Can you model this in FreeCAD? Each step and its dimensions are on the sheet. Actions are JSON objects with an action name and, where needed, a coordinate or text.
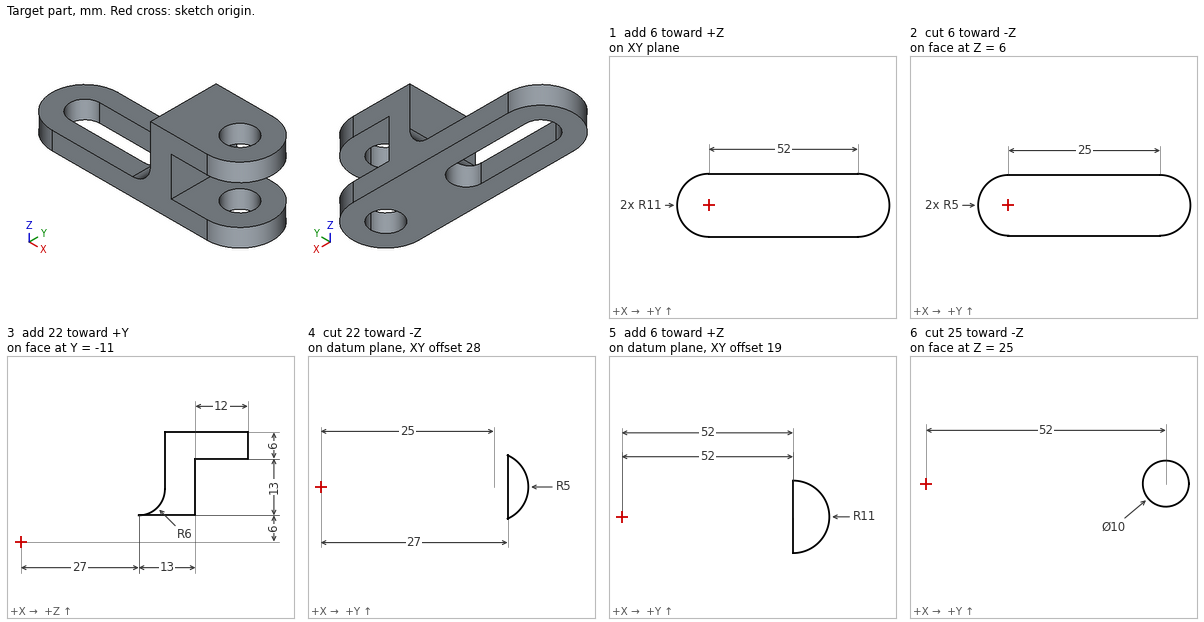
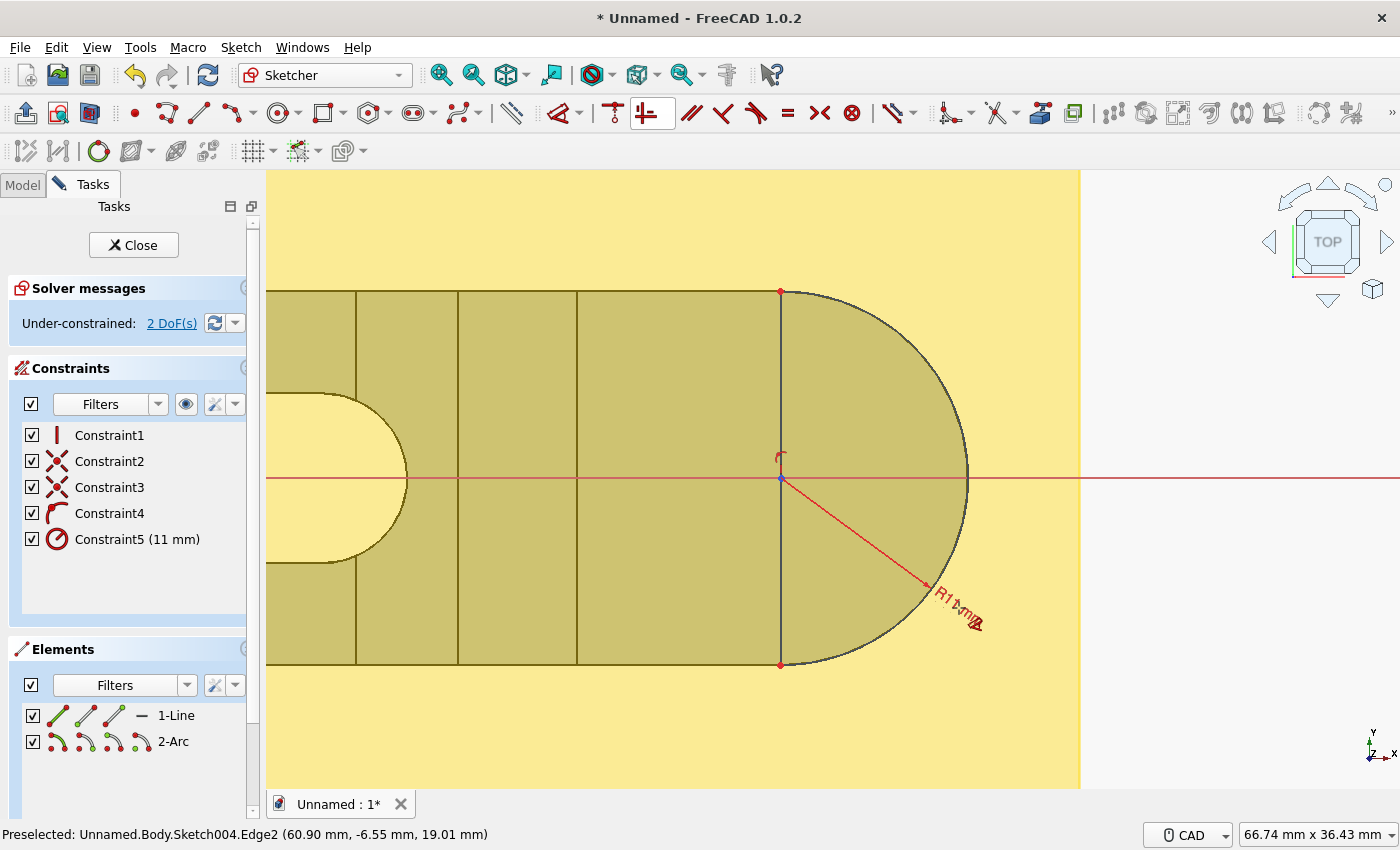
{"action": "left_click", "coordinate": [781, 291]}
{"action": "left_click", "coordinate": [537, 257]}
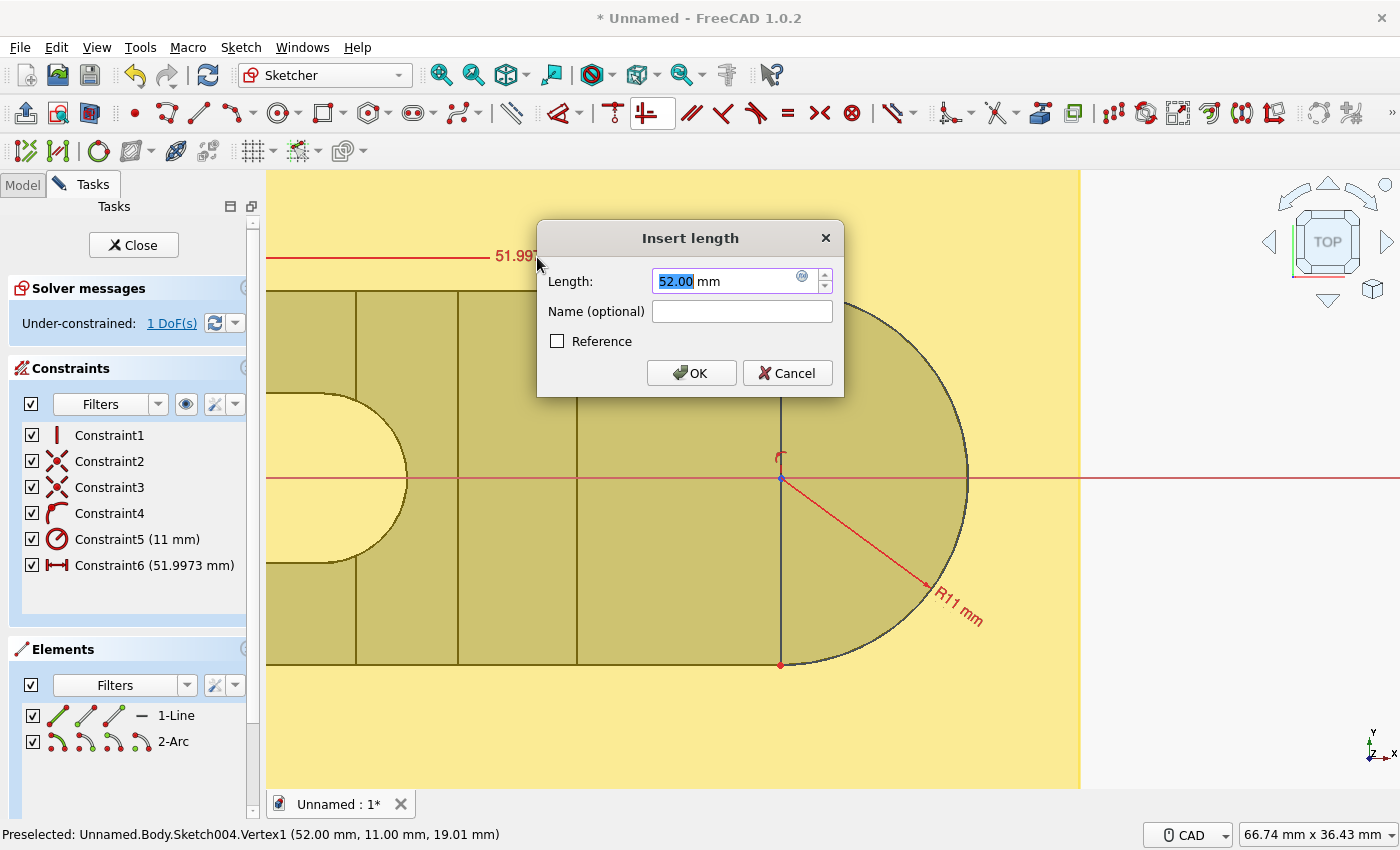
{"action": "type", "text": "52"}
{"action": "key", "text": "Return"}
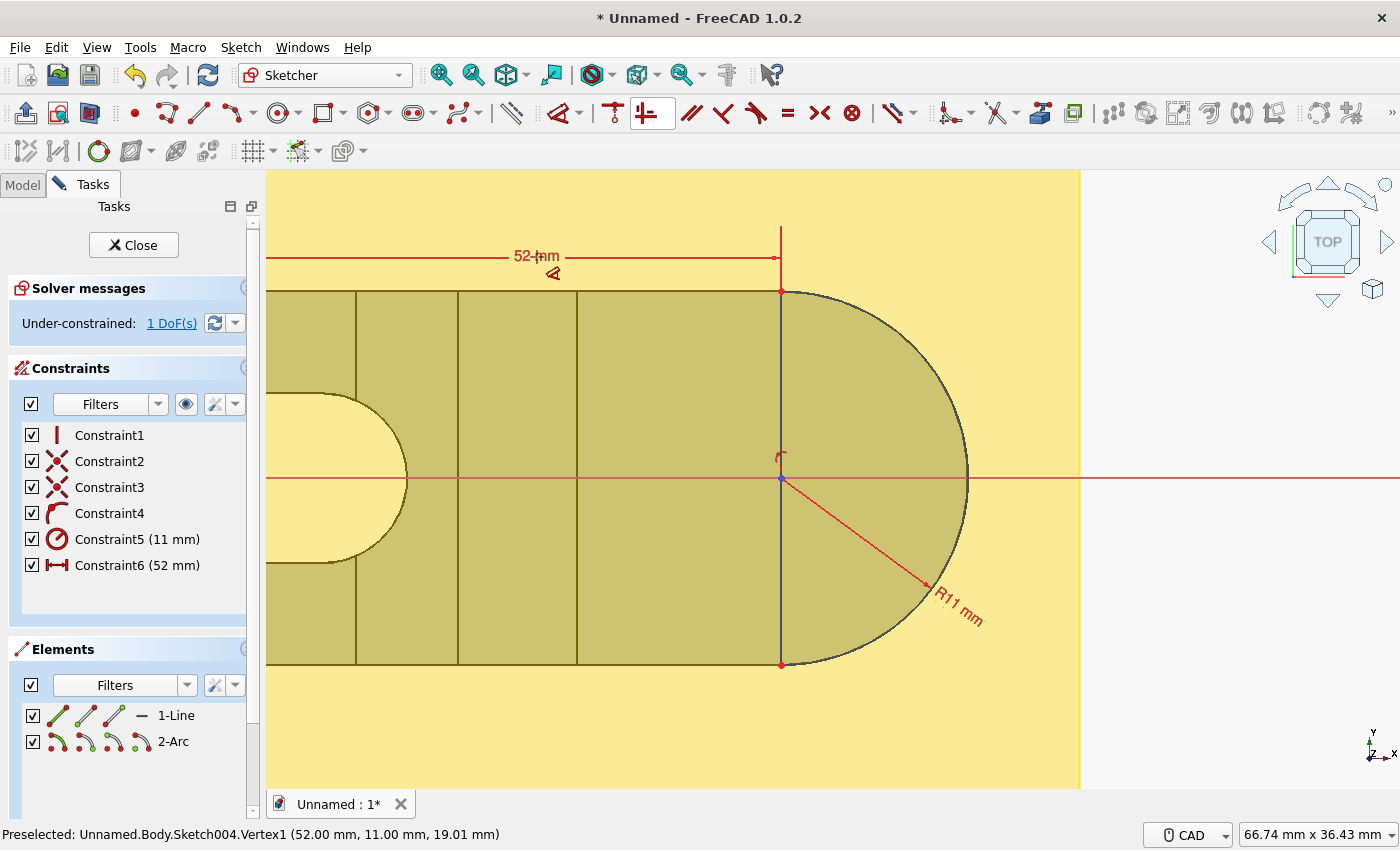
{"action": "left_click", "coordinate": [781, 478]}
{"action": "left_click", "coordinate": [538, 512]}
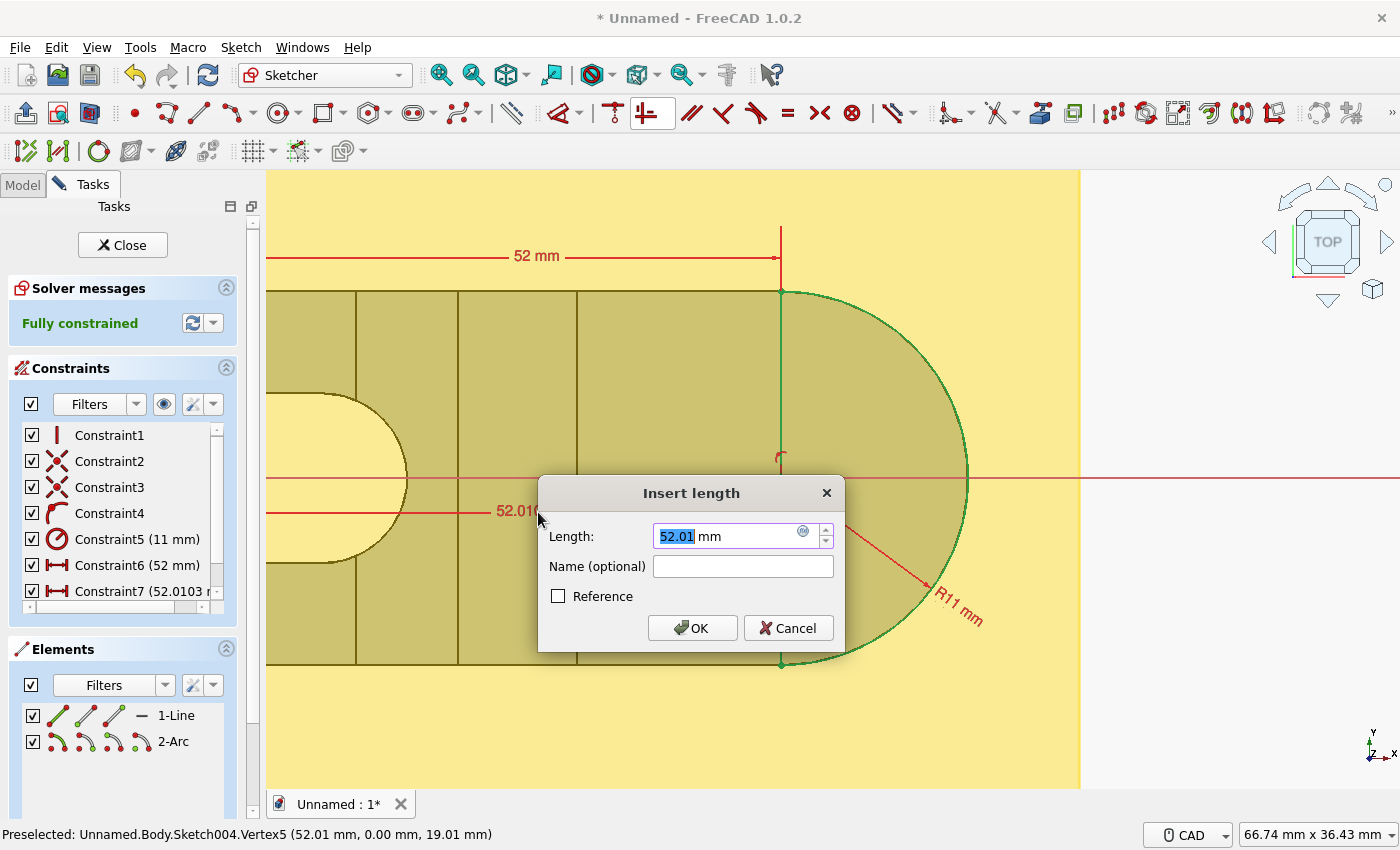
{"action": "type", "text": "52"}
{"action": "key", "text": "Return"}
{"action": "key", "text": "Escape"}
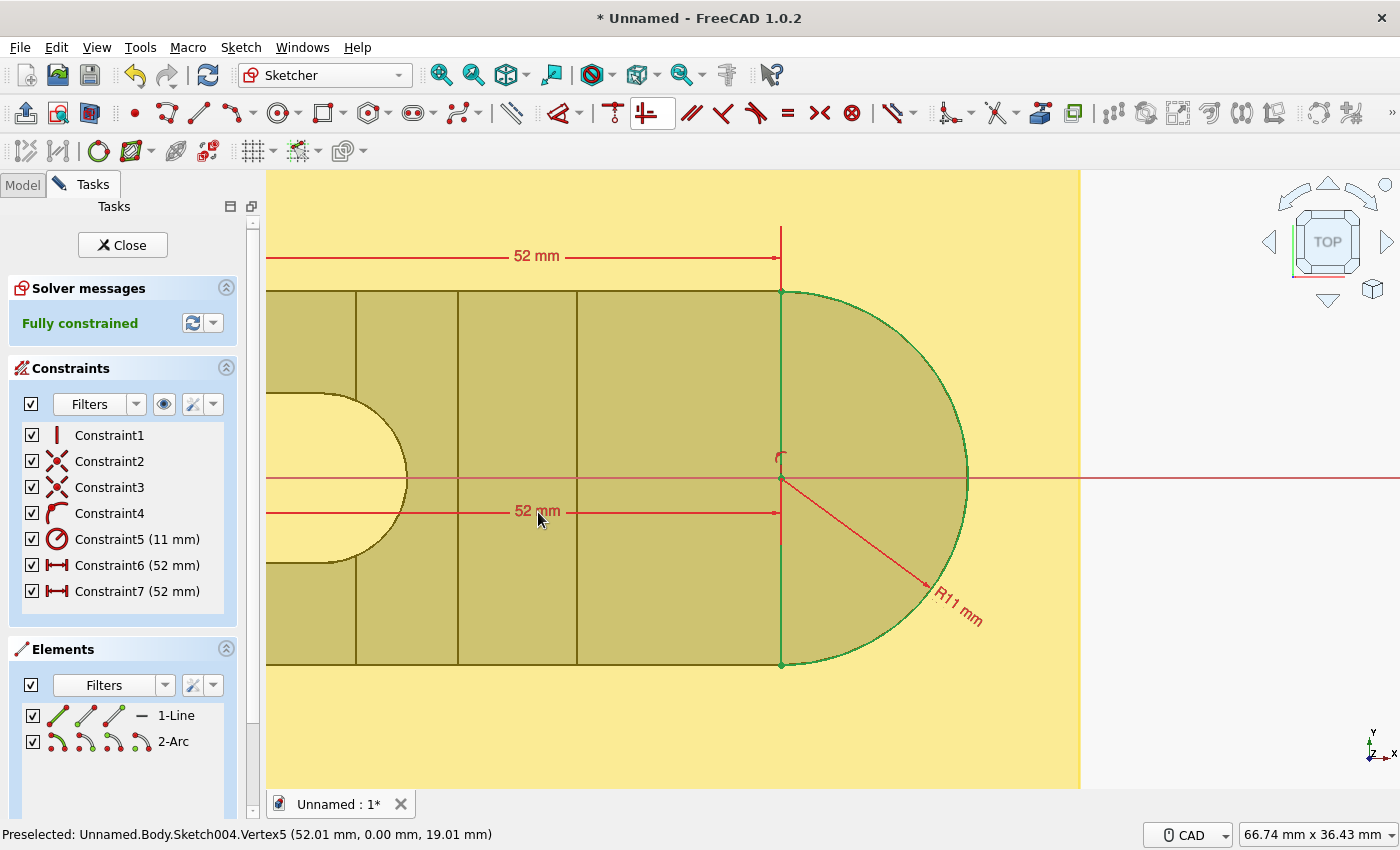
{"action": "left_click", "coordinate": [123, 245]}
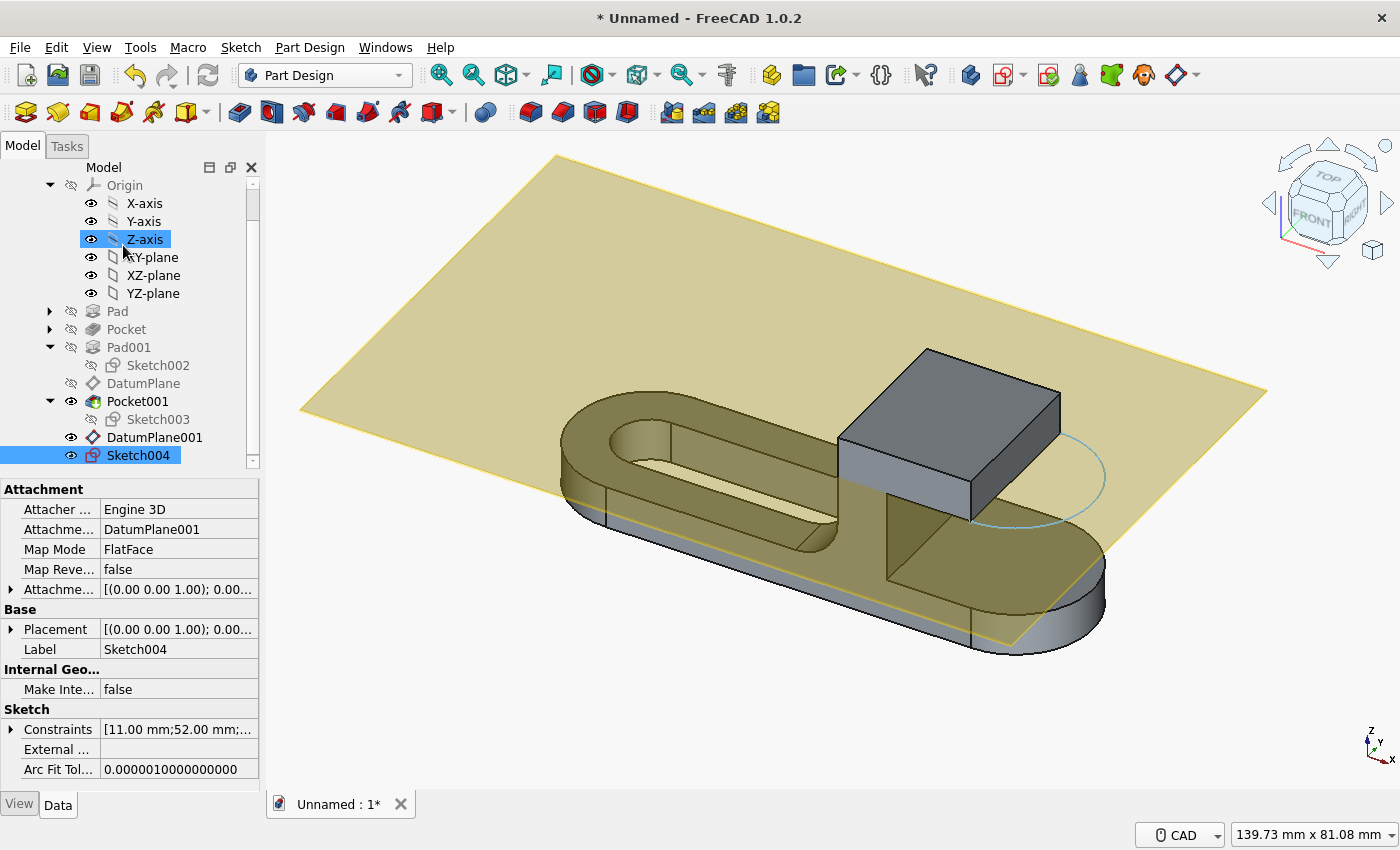
{"action": "left_click", "coordinate": [26, 112]}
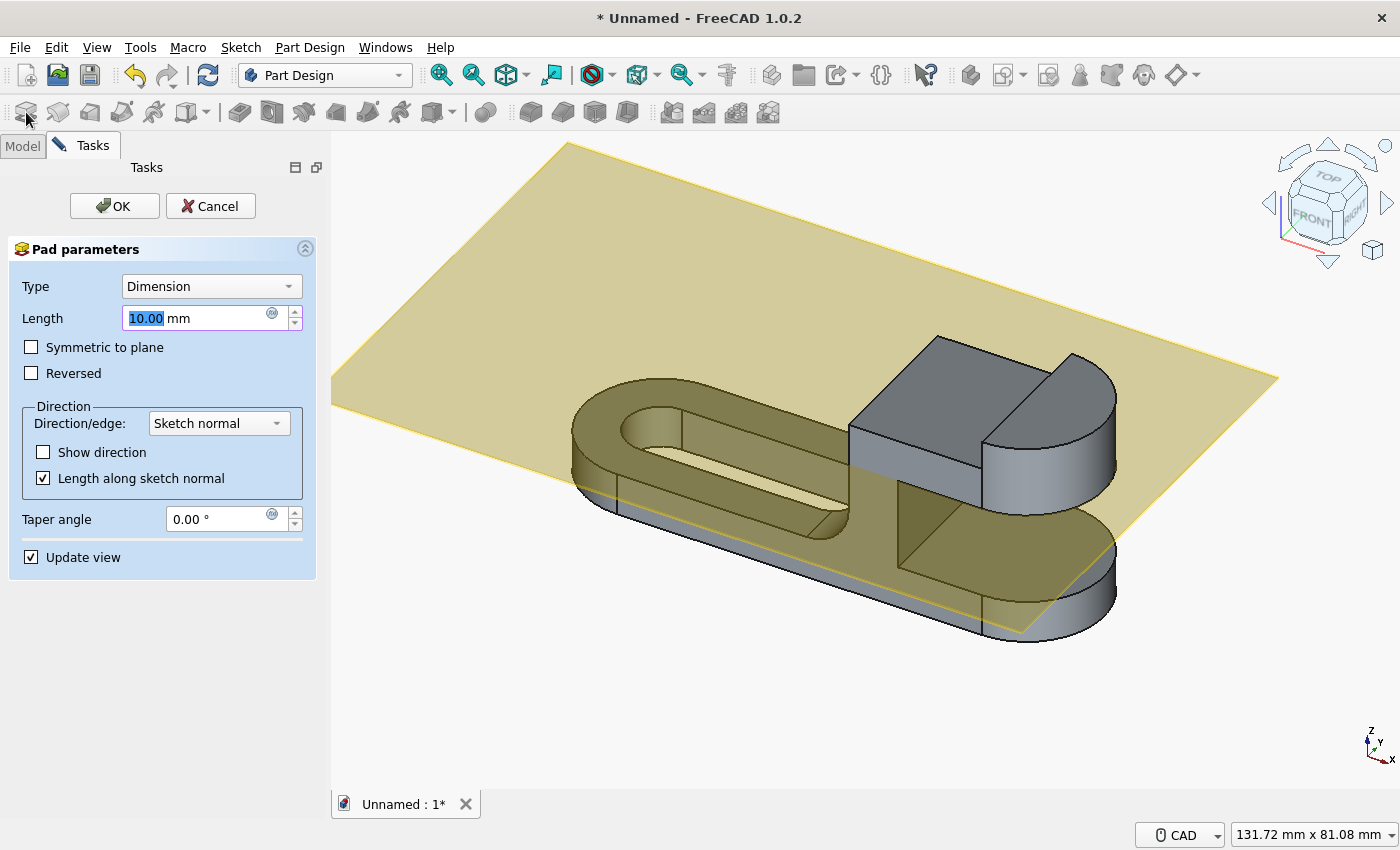
{"action": "type", "text": "6"}
{"action": "key", "text": "Tab"}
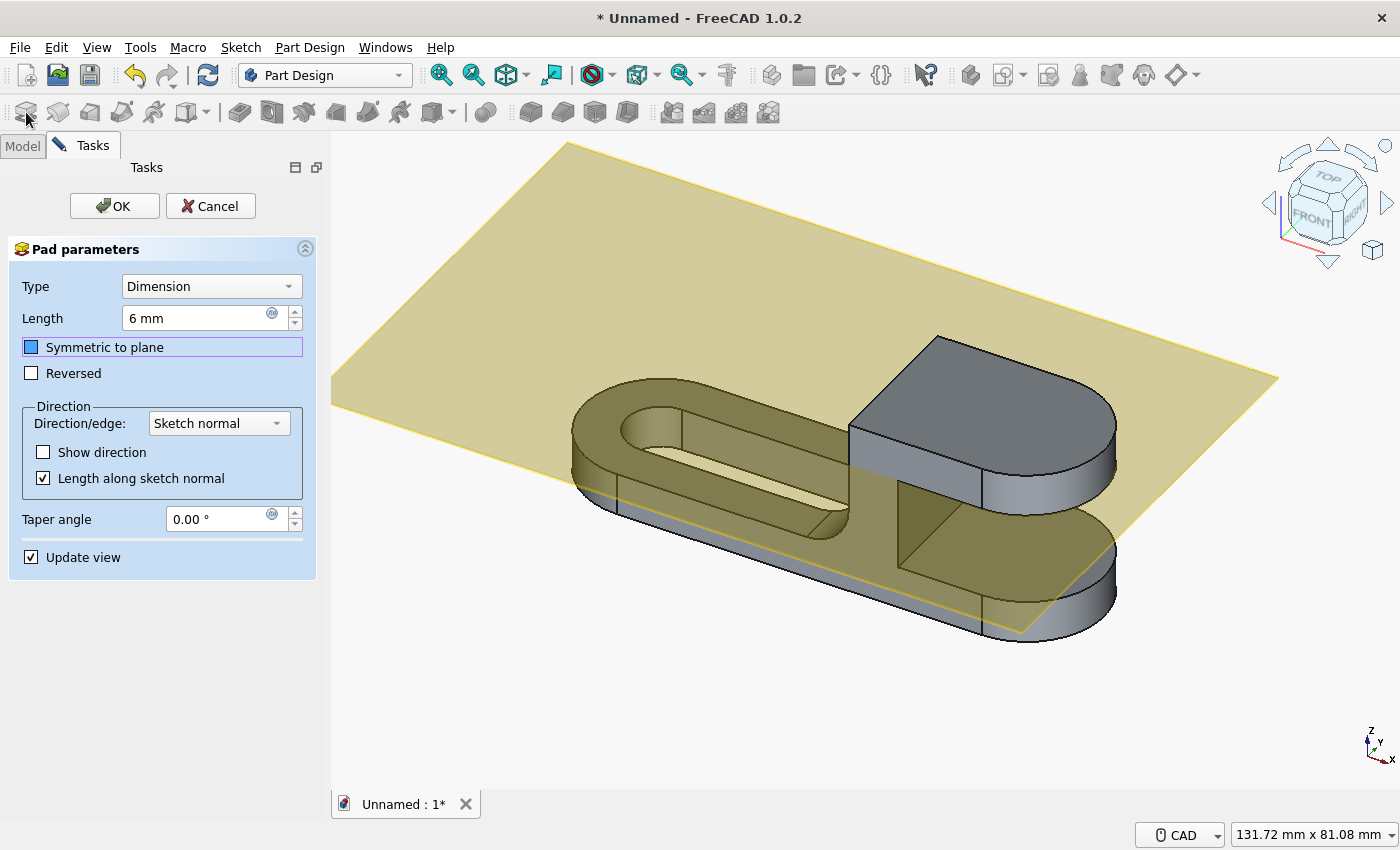
{"action": "left_click", "coordinate": [115, 206]}